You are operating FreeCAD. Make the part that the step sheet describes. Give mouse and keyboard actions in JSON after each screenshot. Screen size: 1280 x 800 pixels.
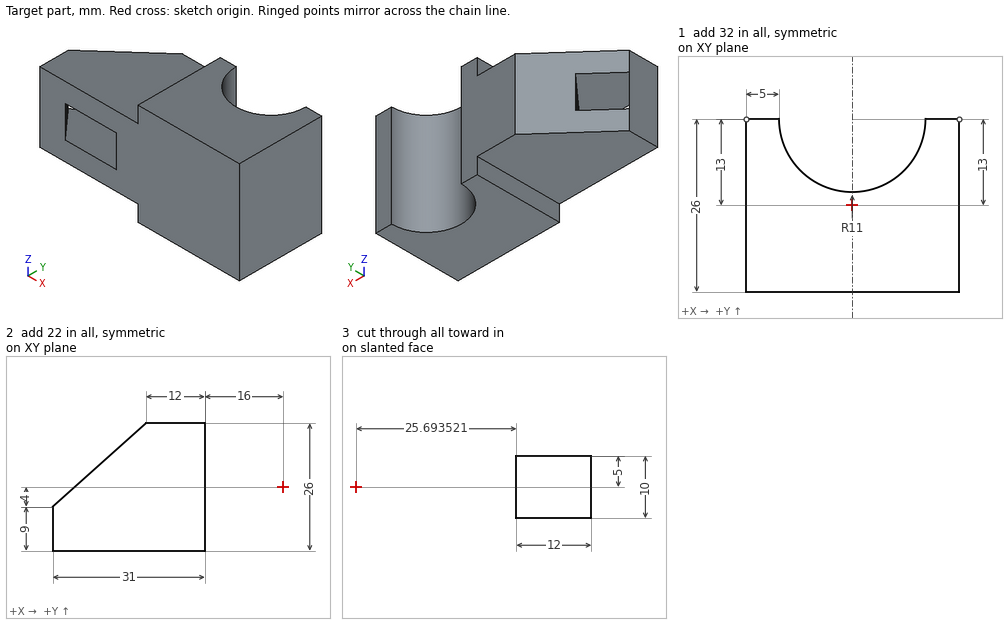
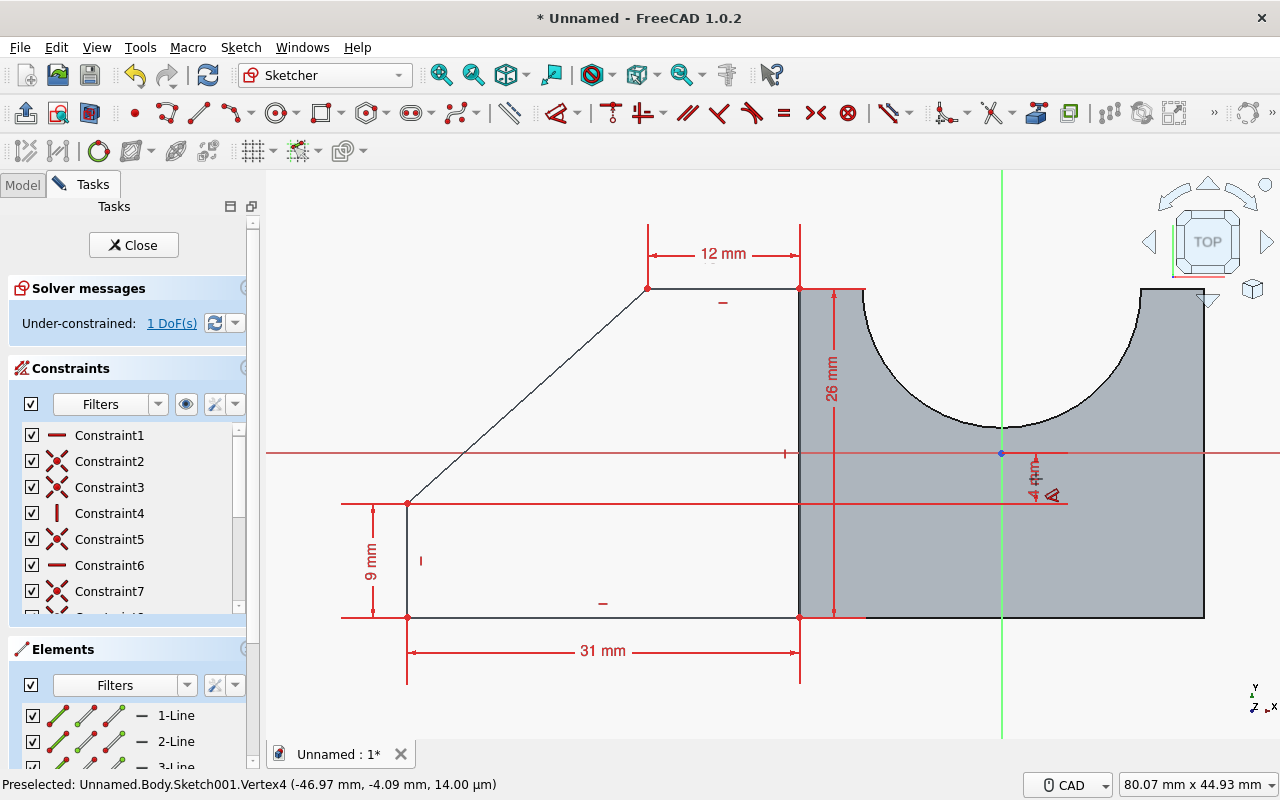
{"action": "left_click", "coordinate": [800, 289]}
{"action": "left_click", "coordinate": [901, 255]}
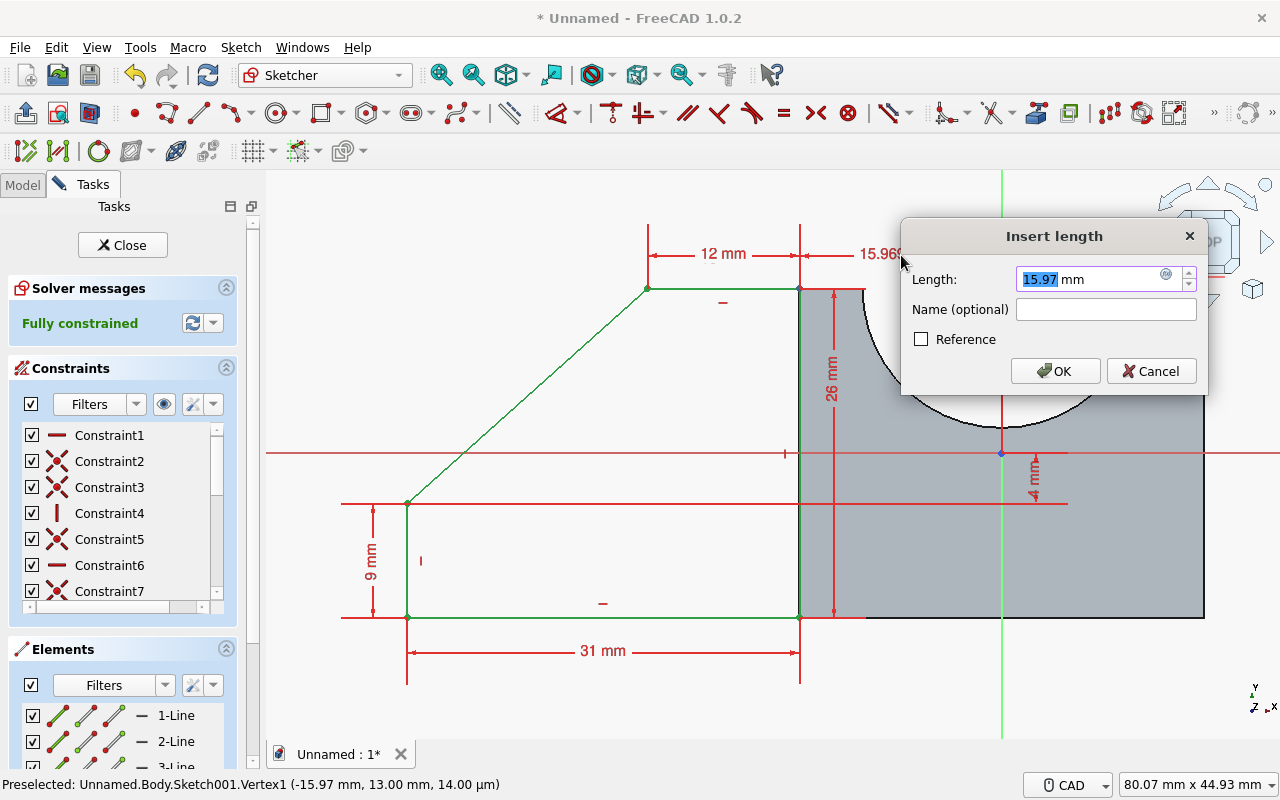
{"action": "type", "text": "16"}
{"action": "key", "text": "Return"}
{"action": "key", "text": "Escape"}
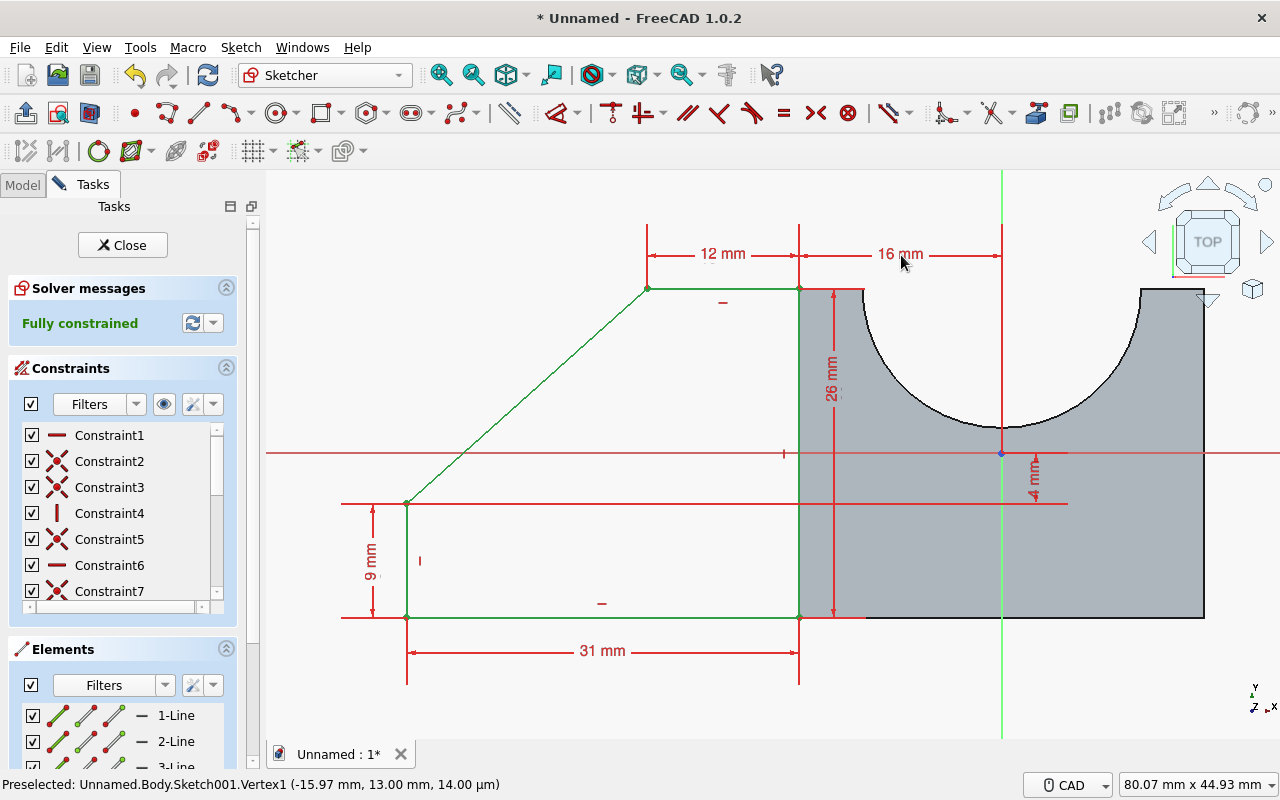
{"action": "left_click", "coordinate": [123, 245]}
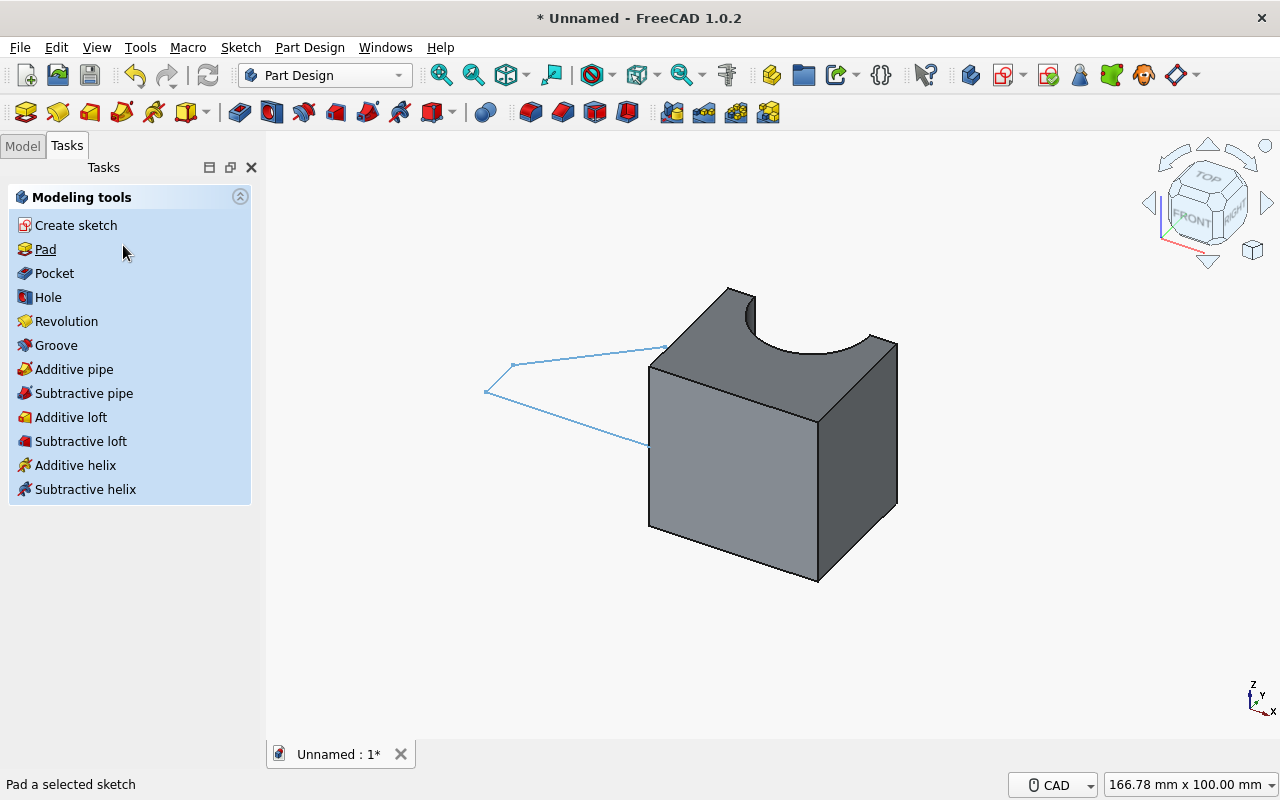
{"action": "left_click", "coordinate": [26, 112]}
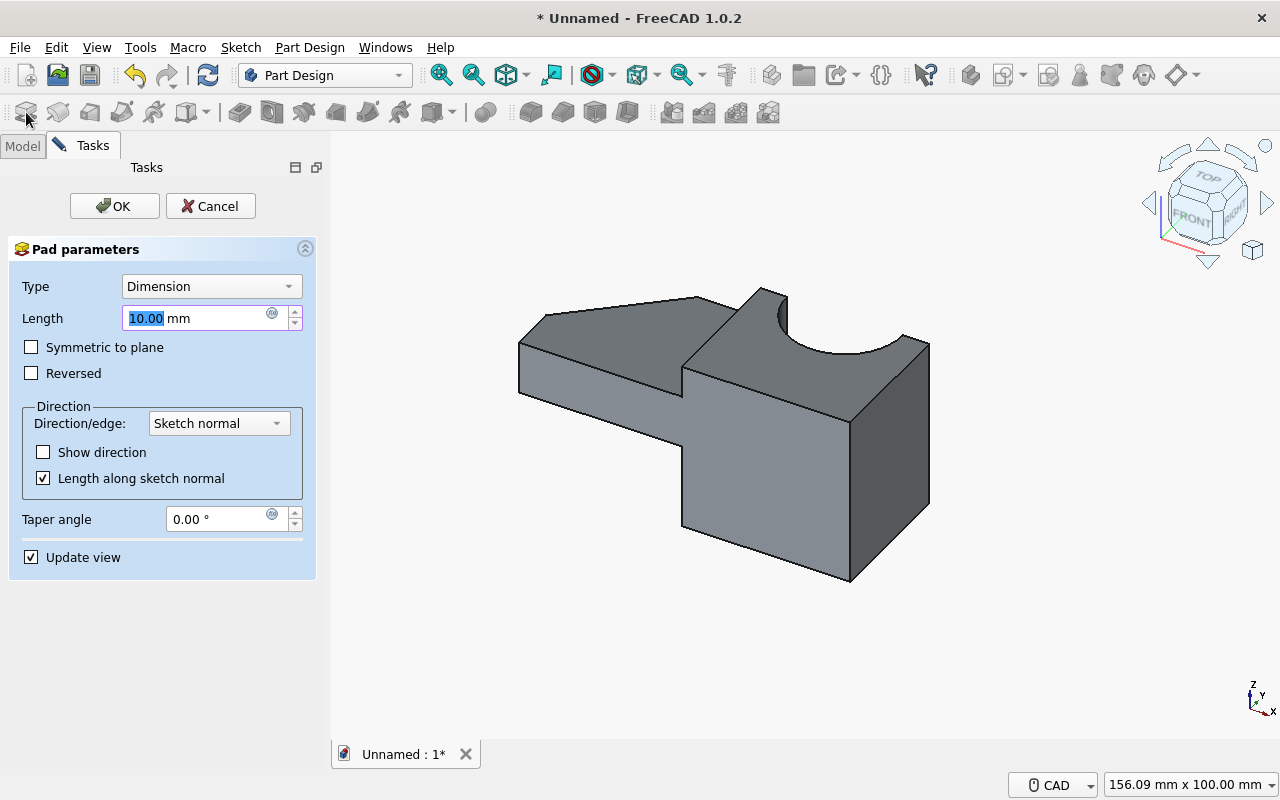
{"action": "type", "text": "22"}
{"action": "key", "text": "Tab"}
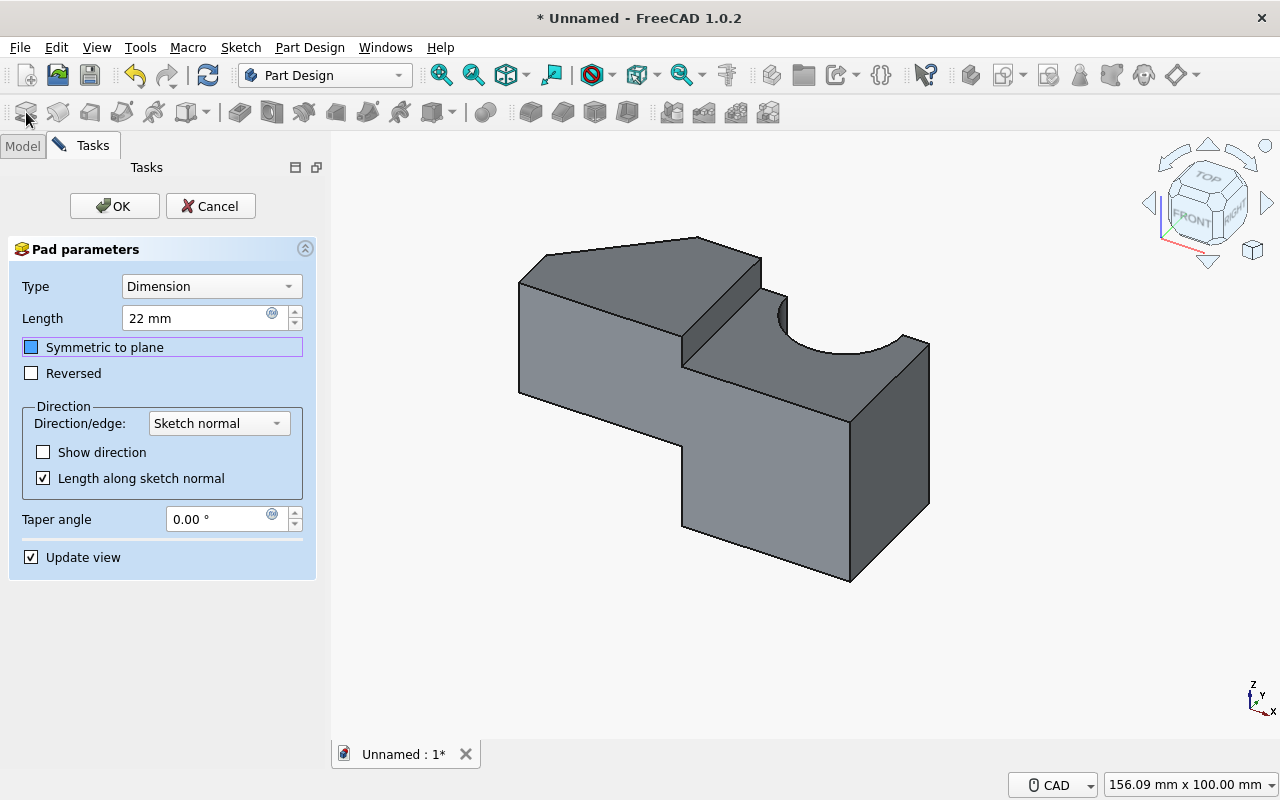
{"action": "left_click", "coordinate": [30, 347]}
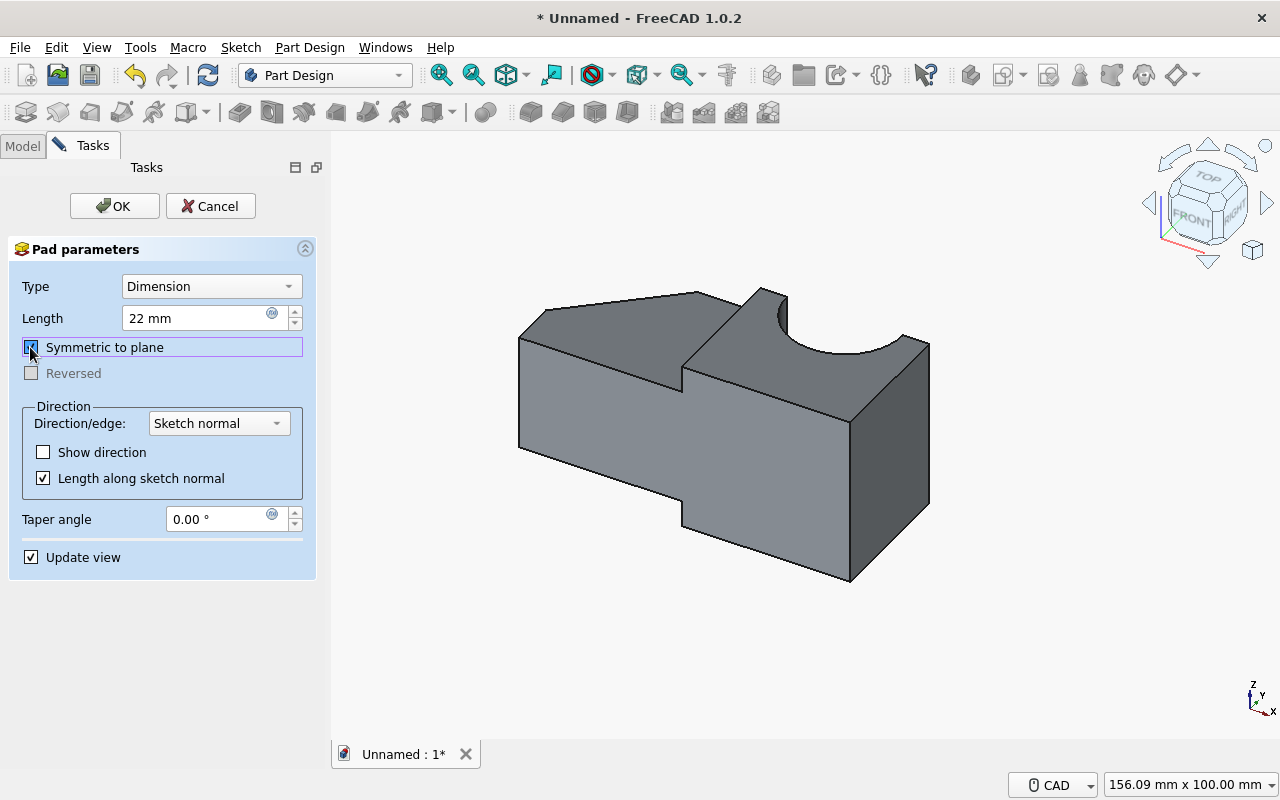
{"action": "left_click", "coordinate": [115, 206]}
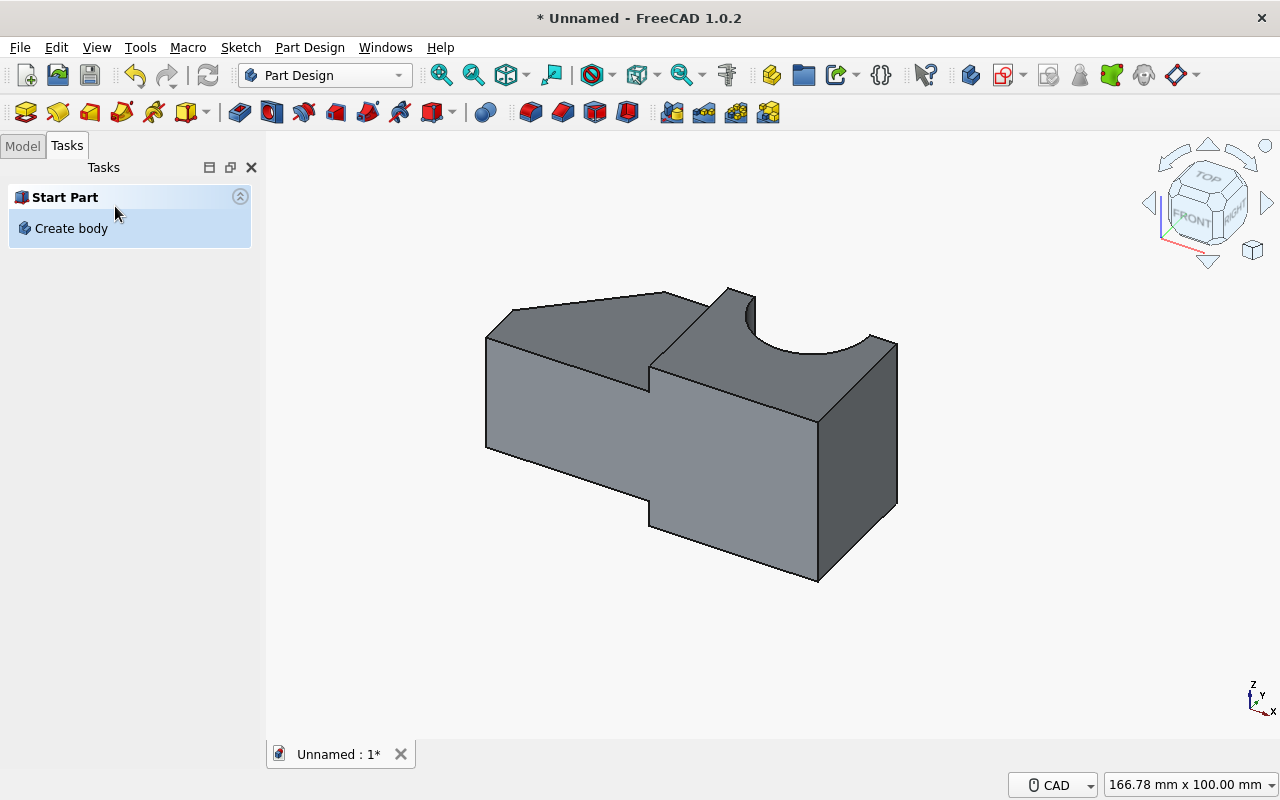
{"action": "key", "text": "4"}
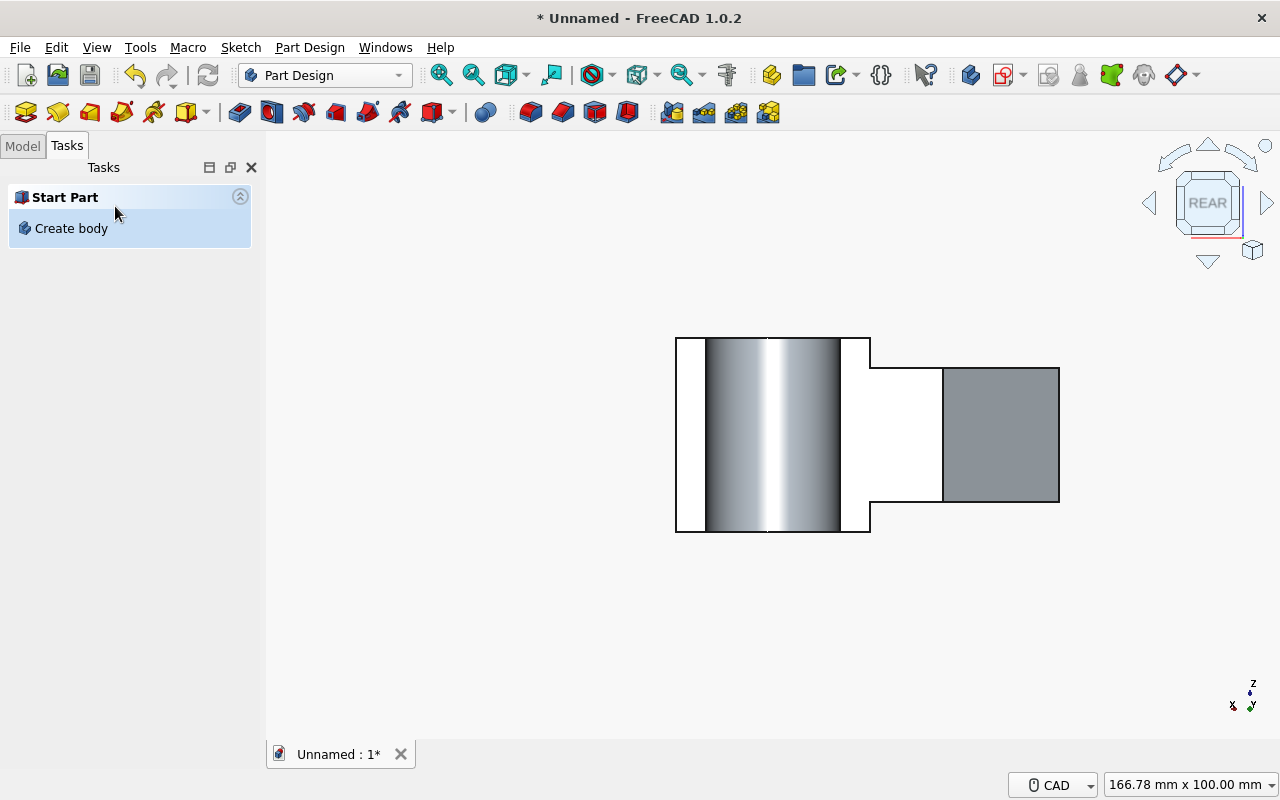
{"action": "key", "text": "v f"}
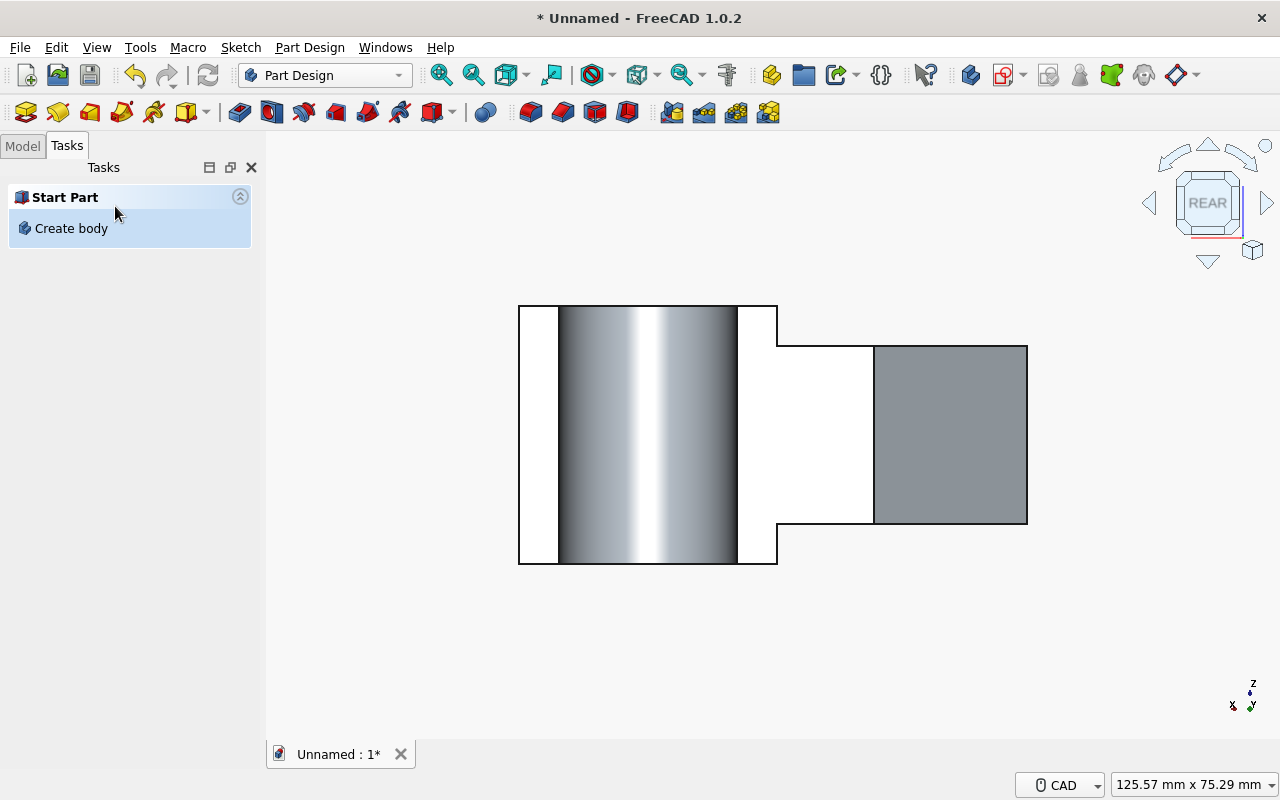
{"action": "left_click", "coordinate": [951, 434]}